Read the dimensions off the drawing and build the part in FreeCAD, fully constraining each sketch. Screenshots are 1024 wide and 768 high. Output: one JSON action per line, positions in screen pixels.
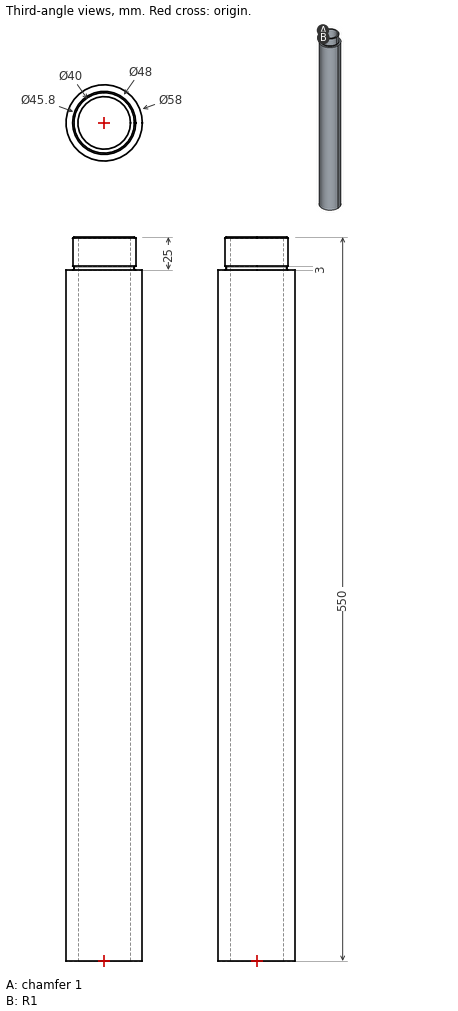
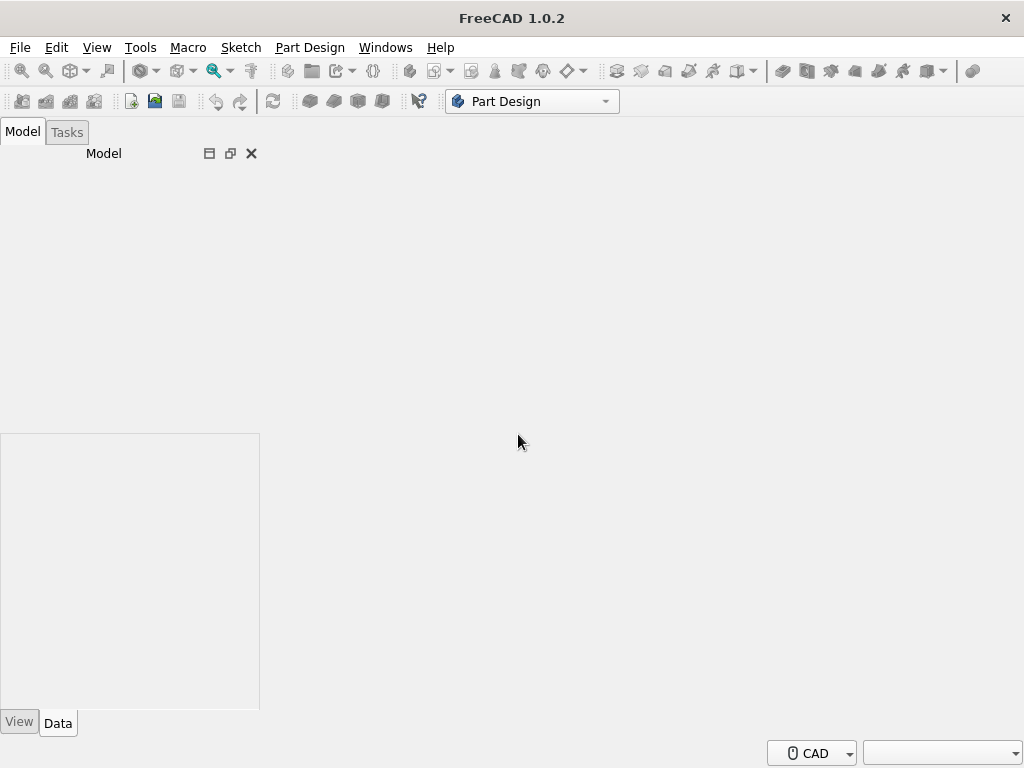
{"action": "left_click", "coordinate": [132, 102]}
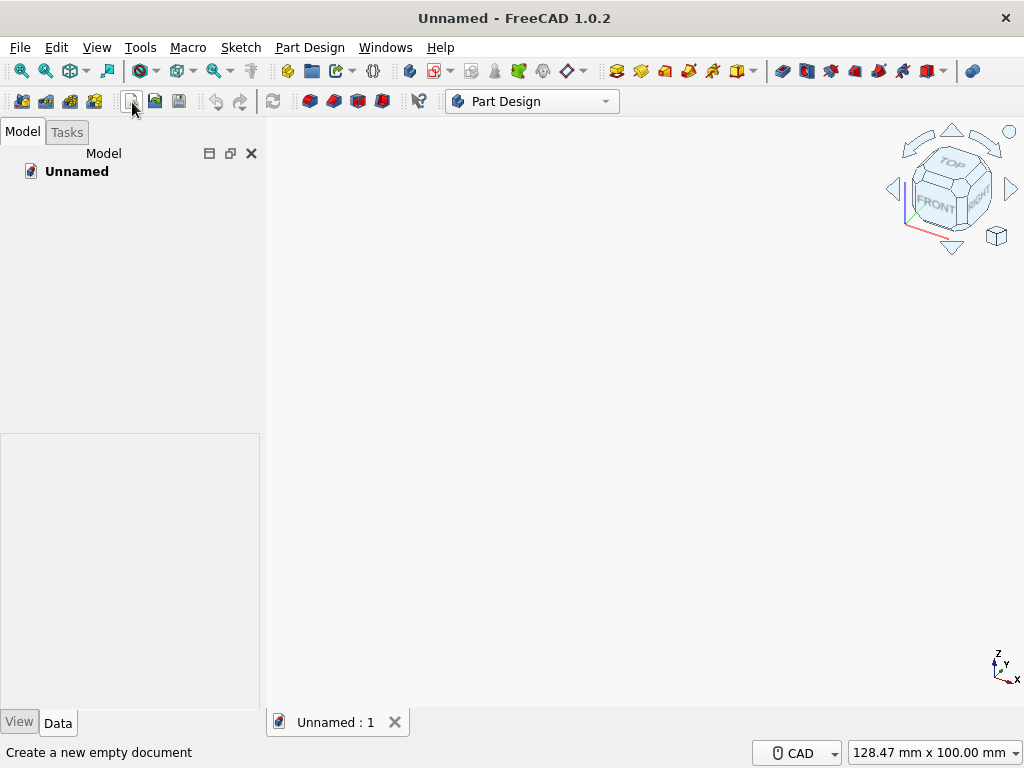
{"action": "left_click", "coordinate": [434, 72]}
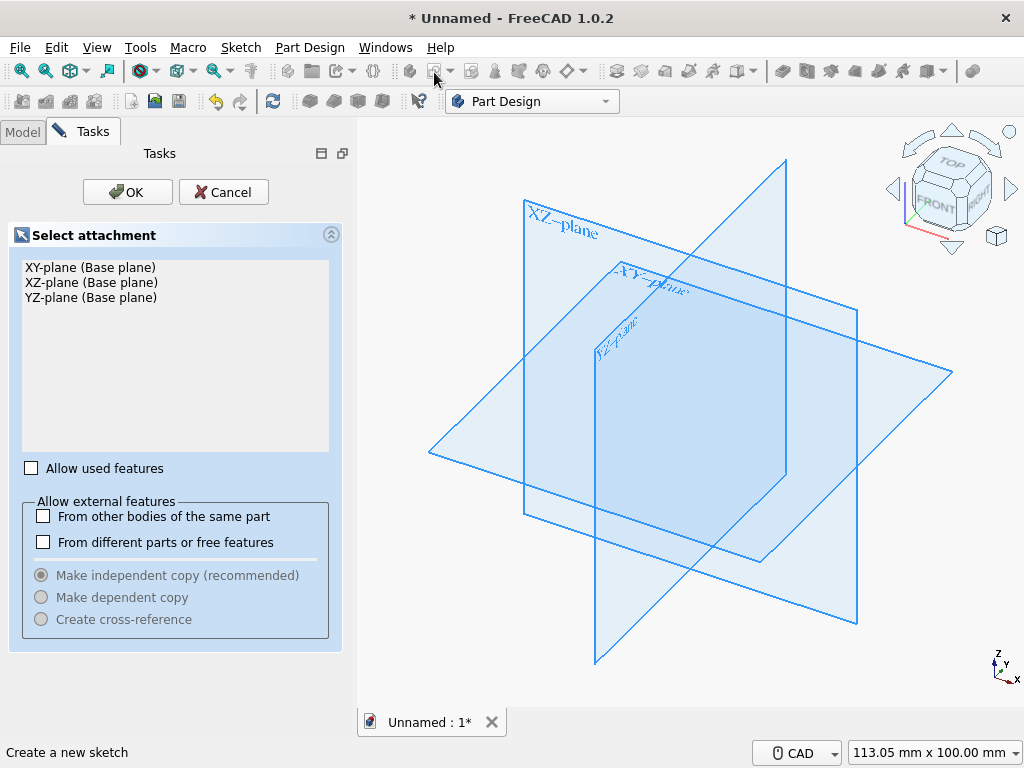
{"action": "left_click", "coordinate": [82, 268]}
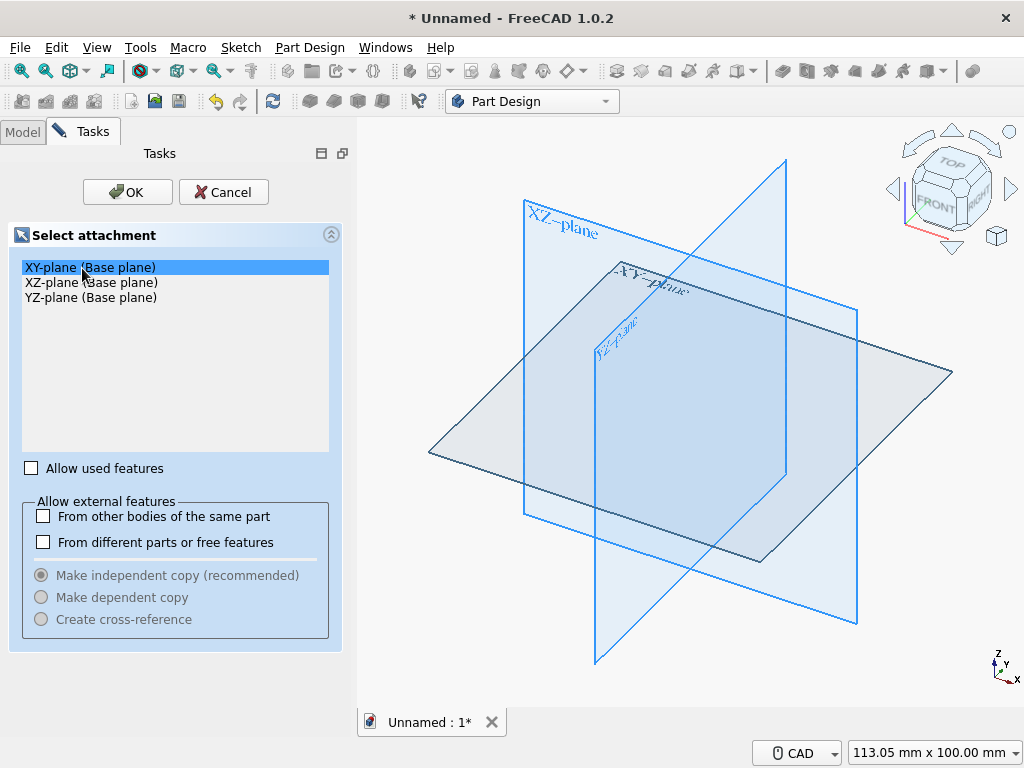
{"action": "left_click", "coordinate": [128, 192]}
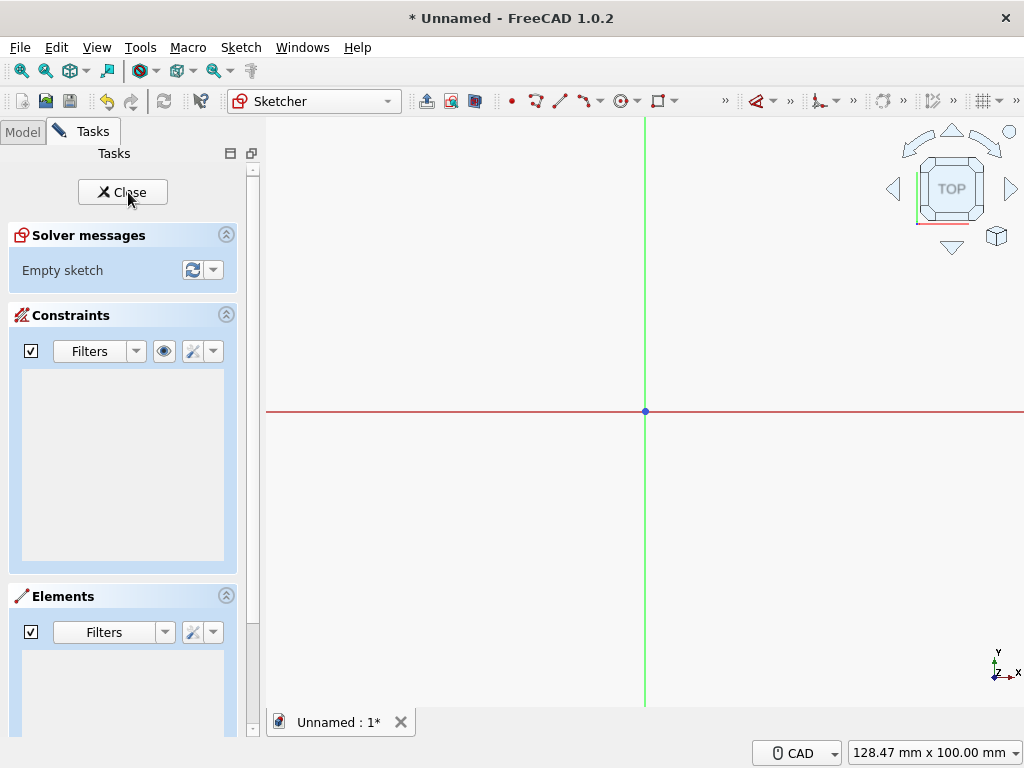
{"action": "left_click", "coordinate": [622, 102]}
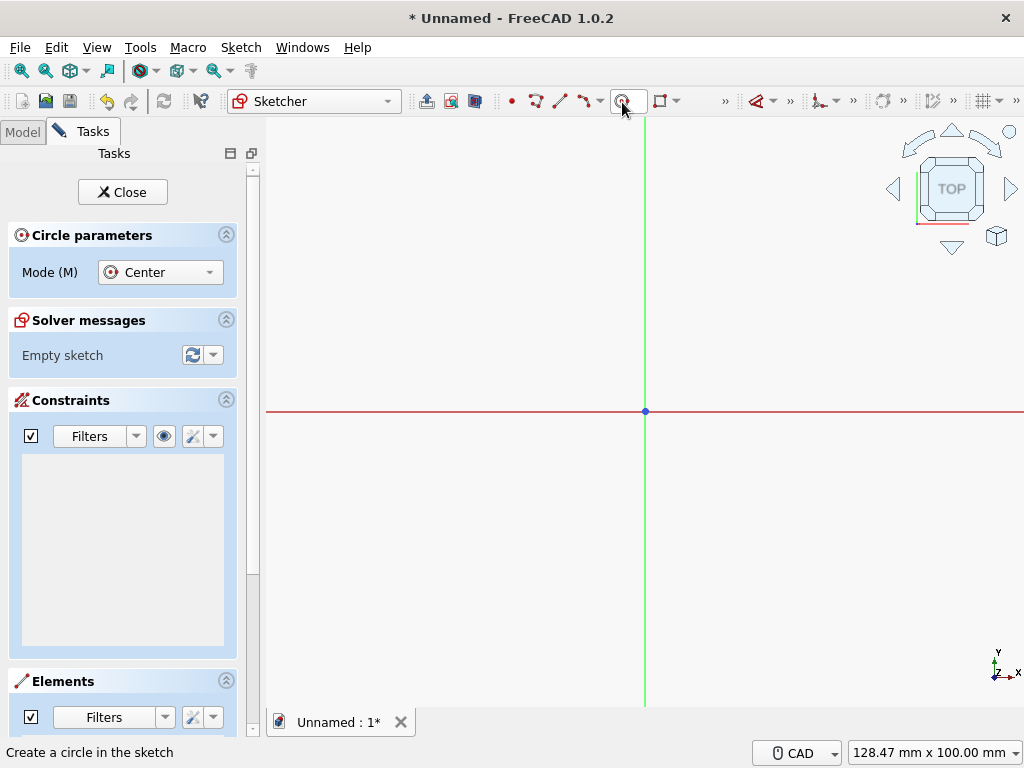
{"action": "left_click", "coordinate": [645, 412]}
{"action": "mouse_move", "coordinate": [766, 291]}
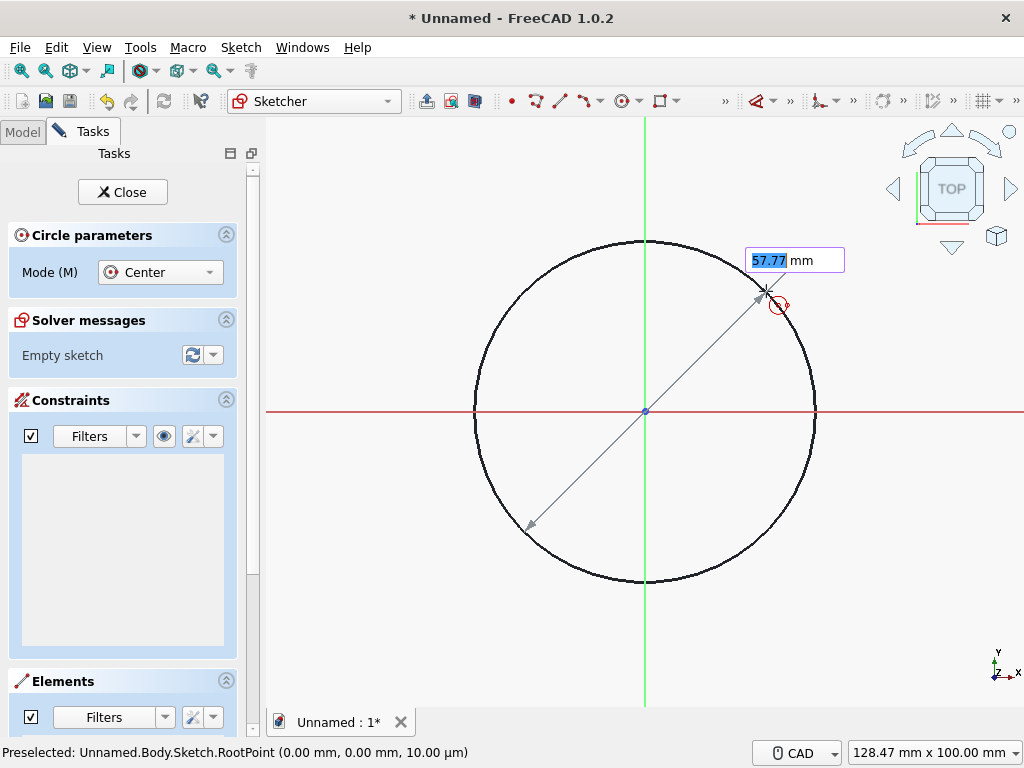
{"action": "type", "text": "58"}
{"action": "key", "text": "Return"}
{"action": "key", "text": "Escape"}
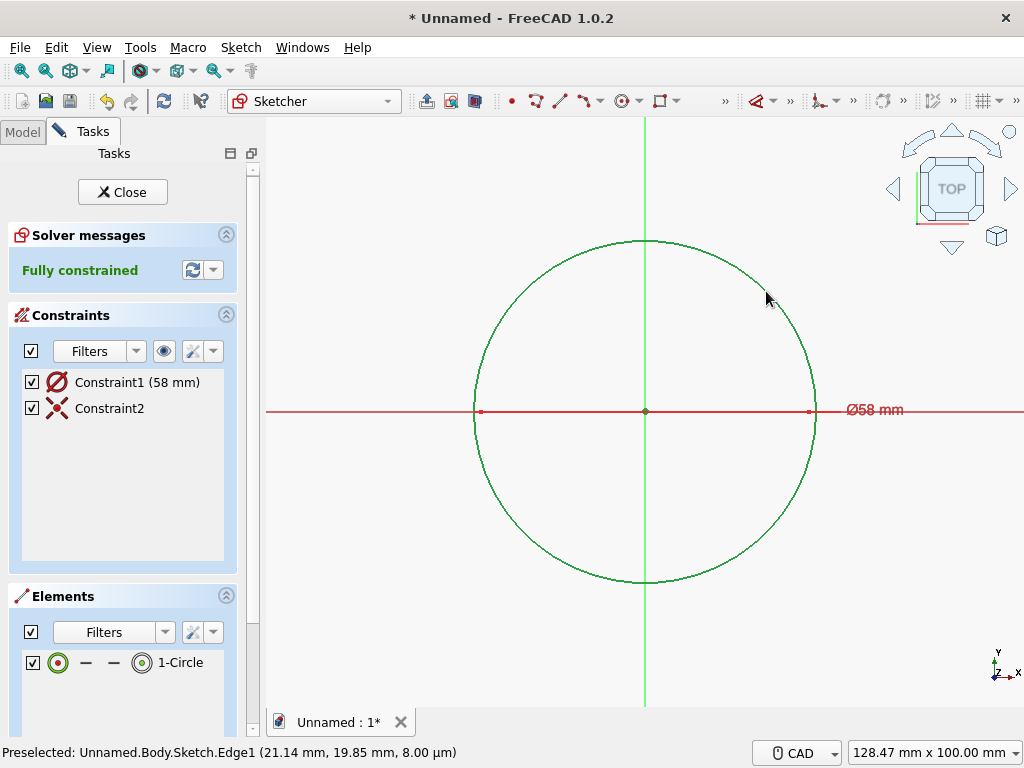
{"action": "left_click", "coordinate": [123, 192]}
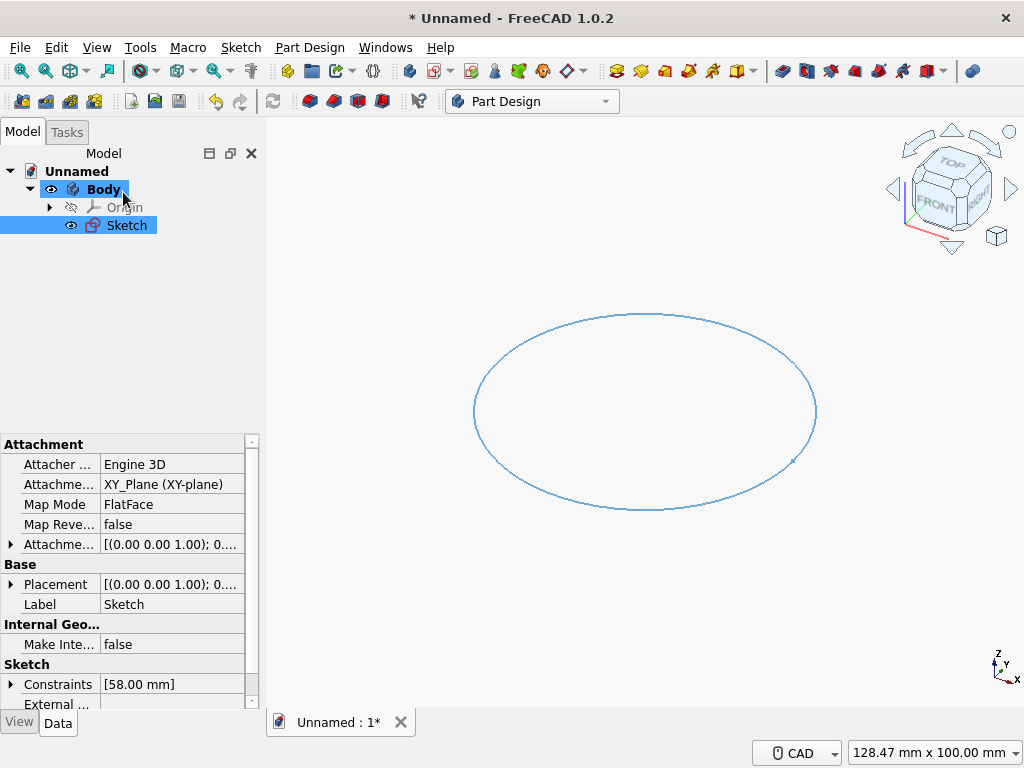
{"action": "left_click", "coordinate": [618, 72]}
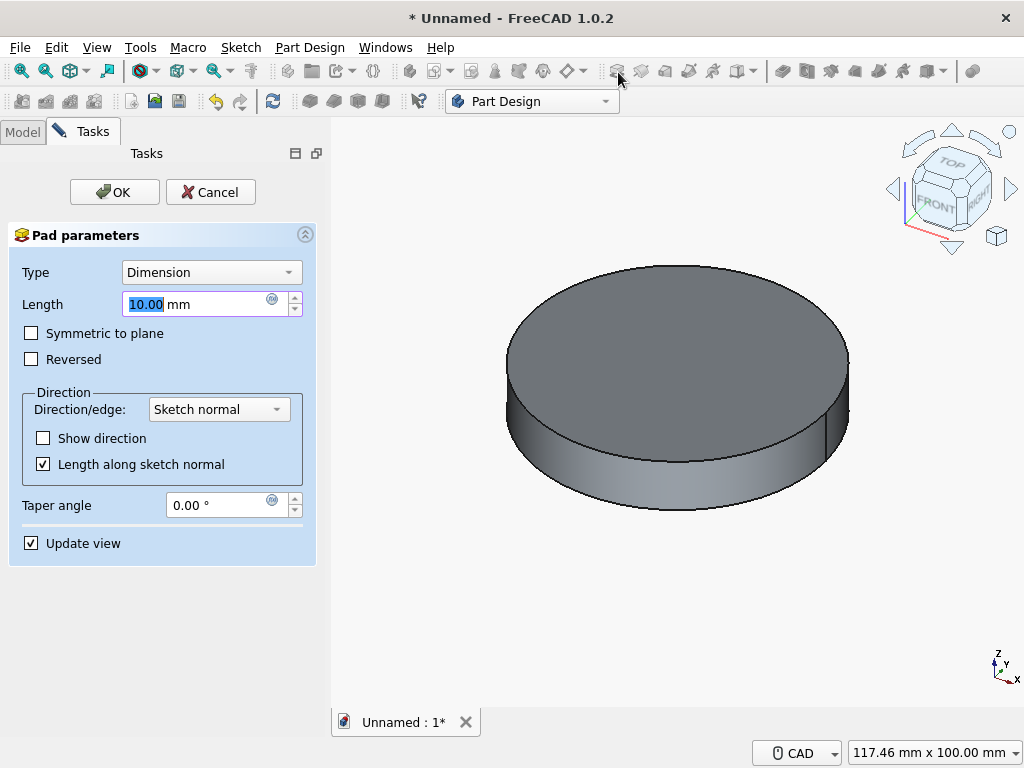
{"action": "type", "text": "550"}
{"action": "key", "text": "Tab"}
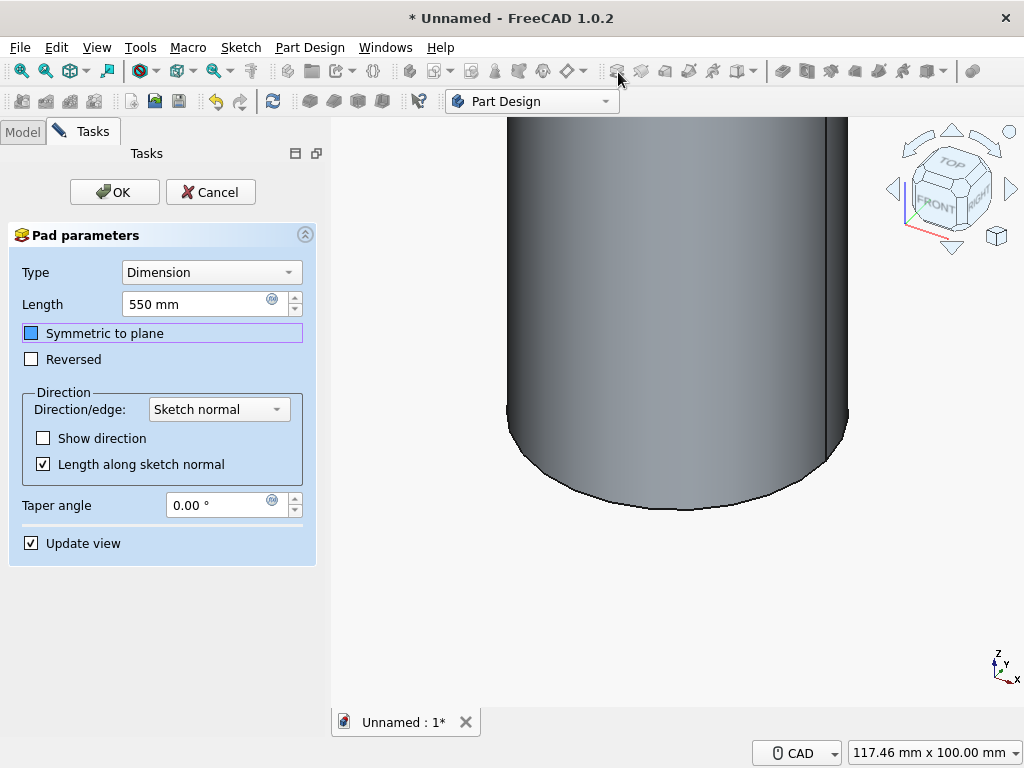
{"action": "left_click", "coordinate": [115, 192]}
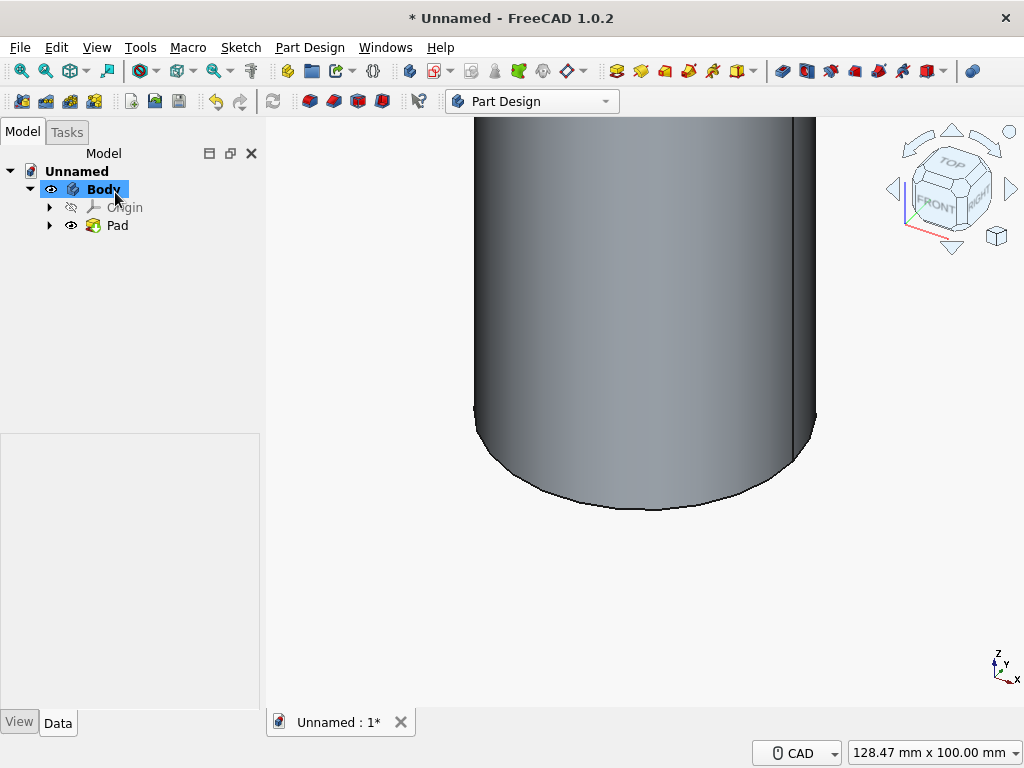
{"action": "left_click", "coordinate": [22, 72]}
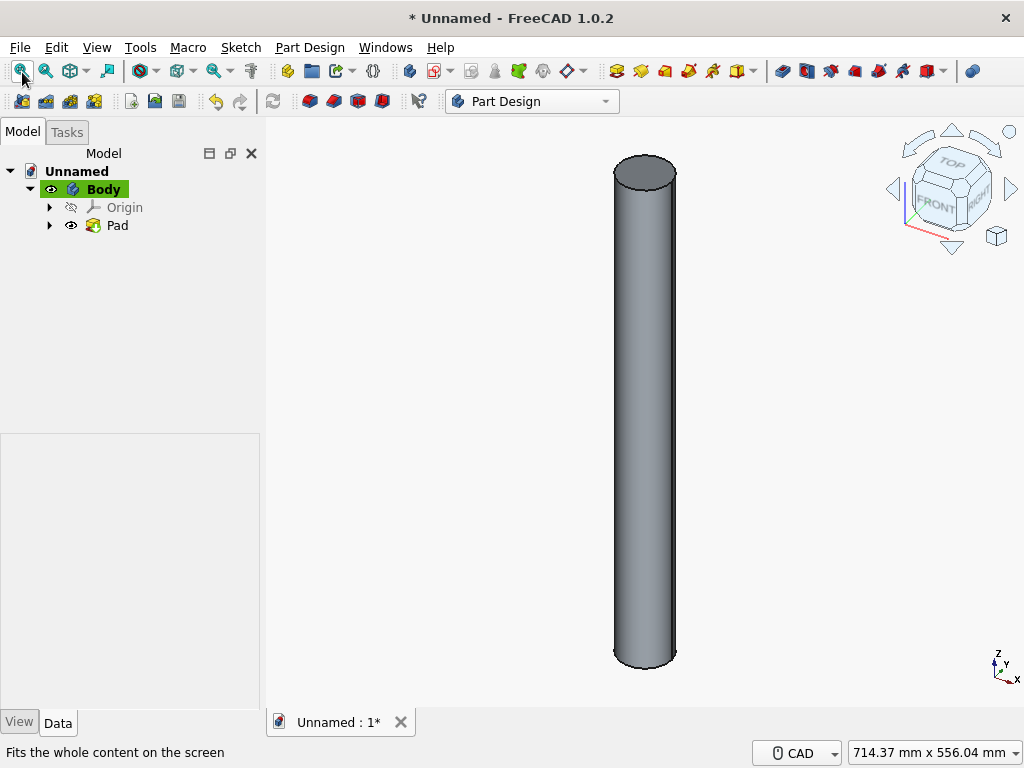
{"action": "left_click", "coordinate": [50, 207]}